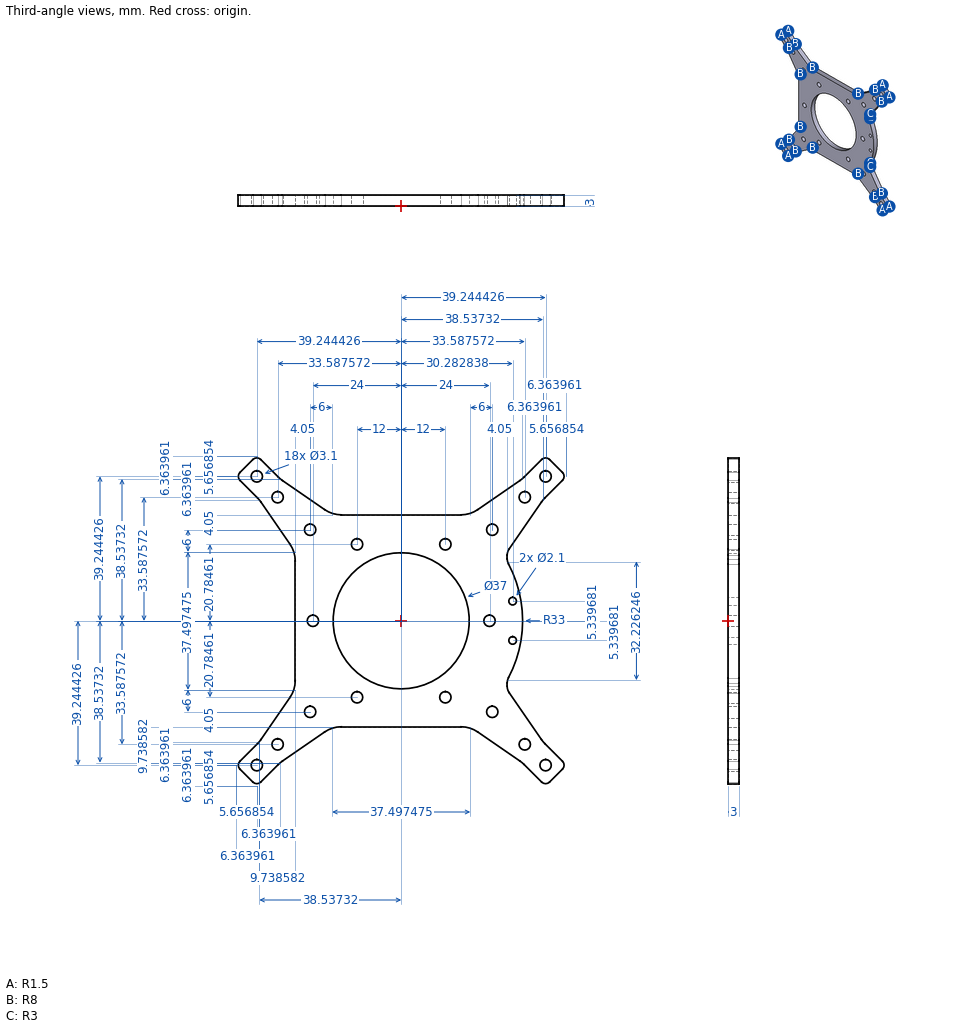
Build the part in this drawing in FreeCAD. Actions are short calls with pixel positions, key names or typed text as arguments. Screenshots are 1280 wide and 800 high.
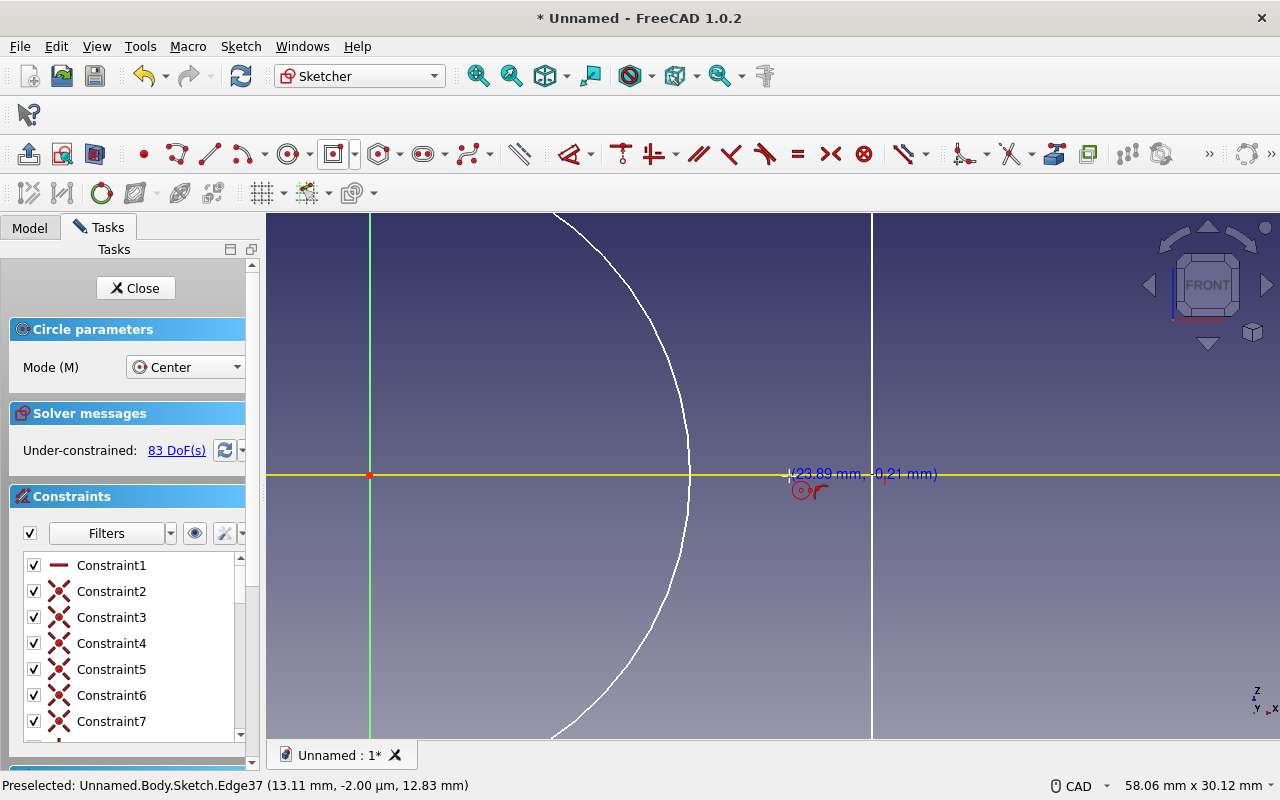
scroll(789, 476, down, 8)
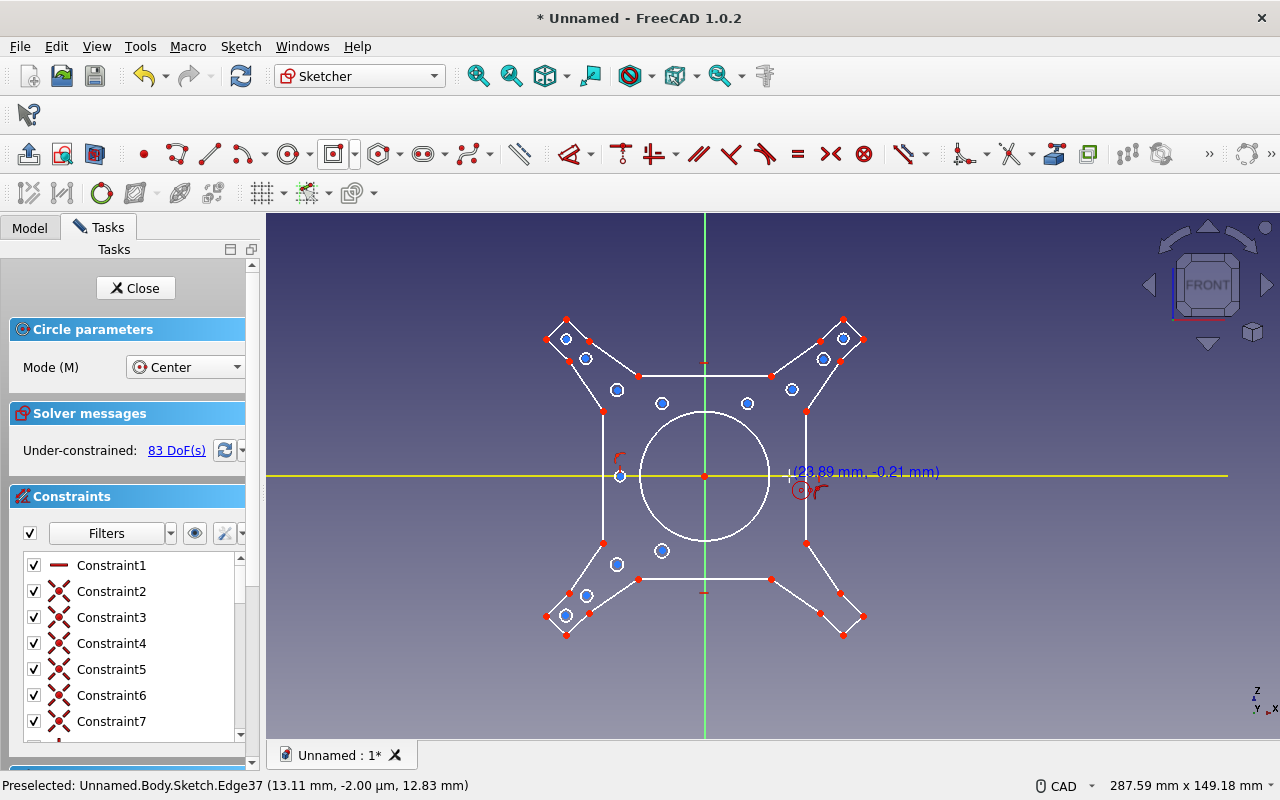
click(789, 476)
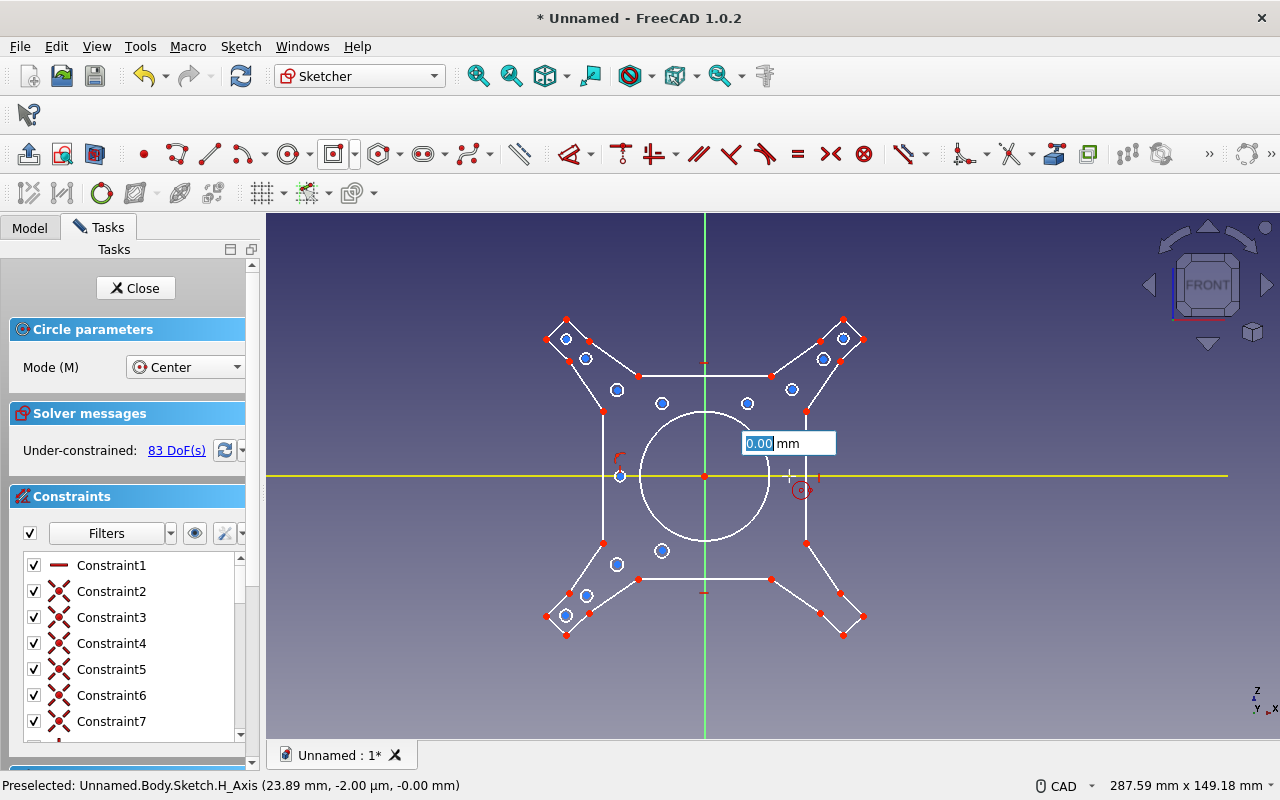
scroll(791, 471, up, 6)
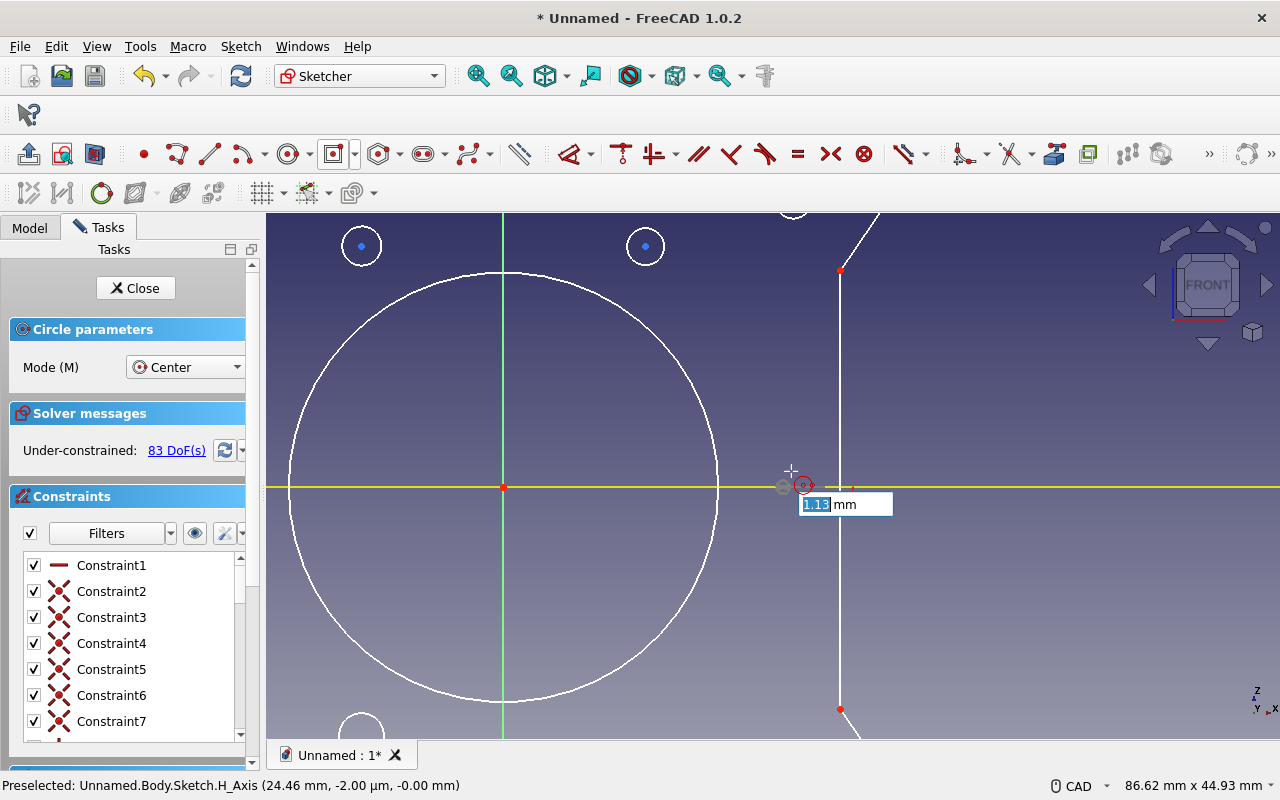
click(791, 470)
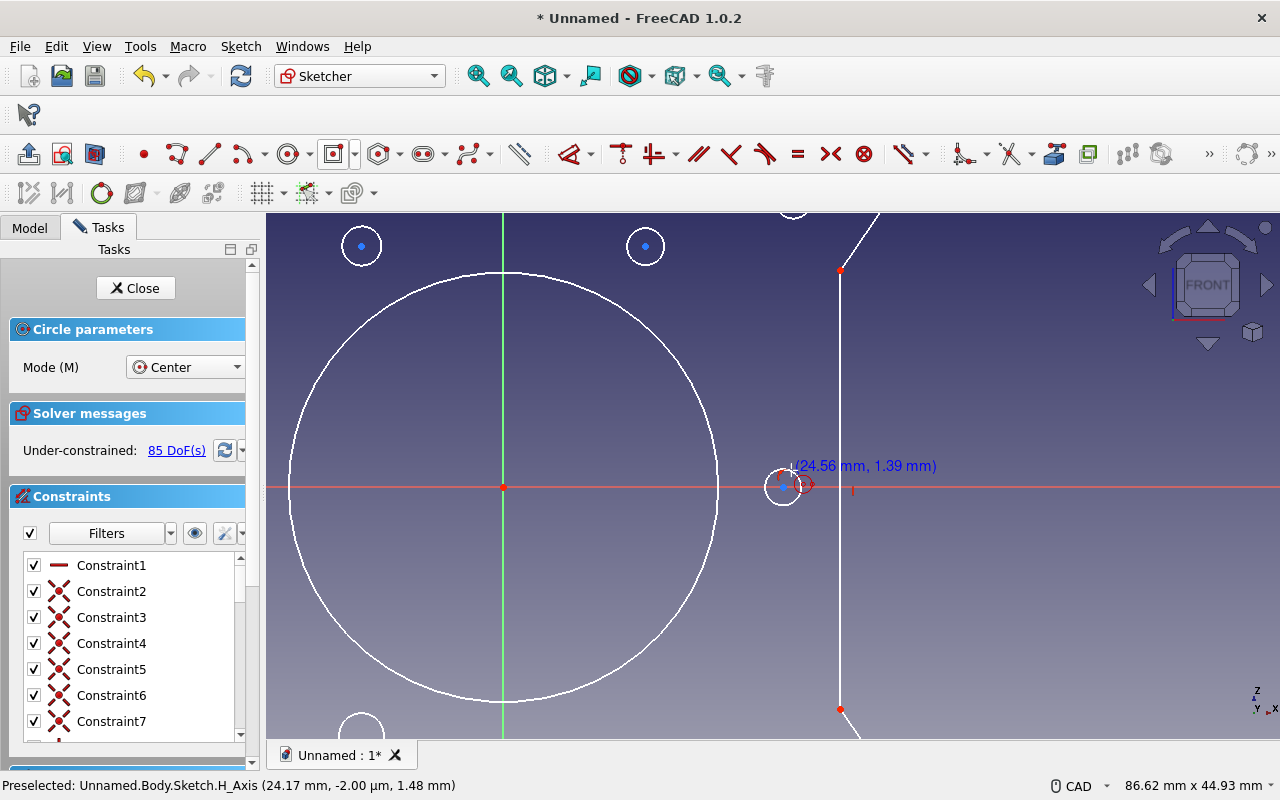
scroll(791, 471, down, 6)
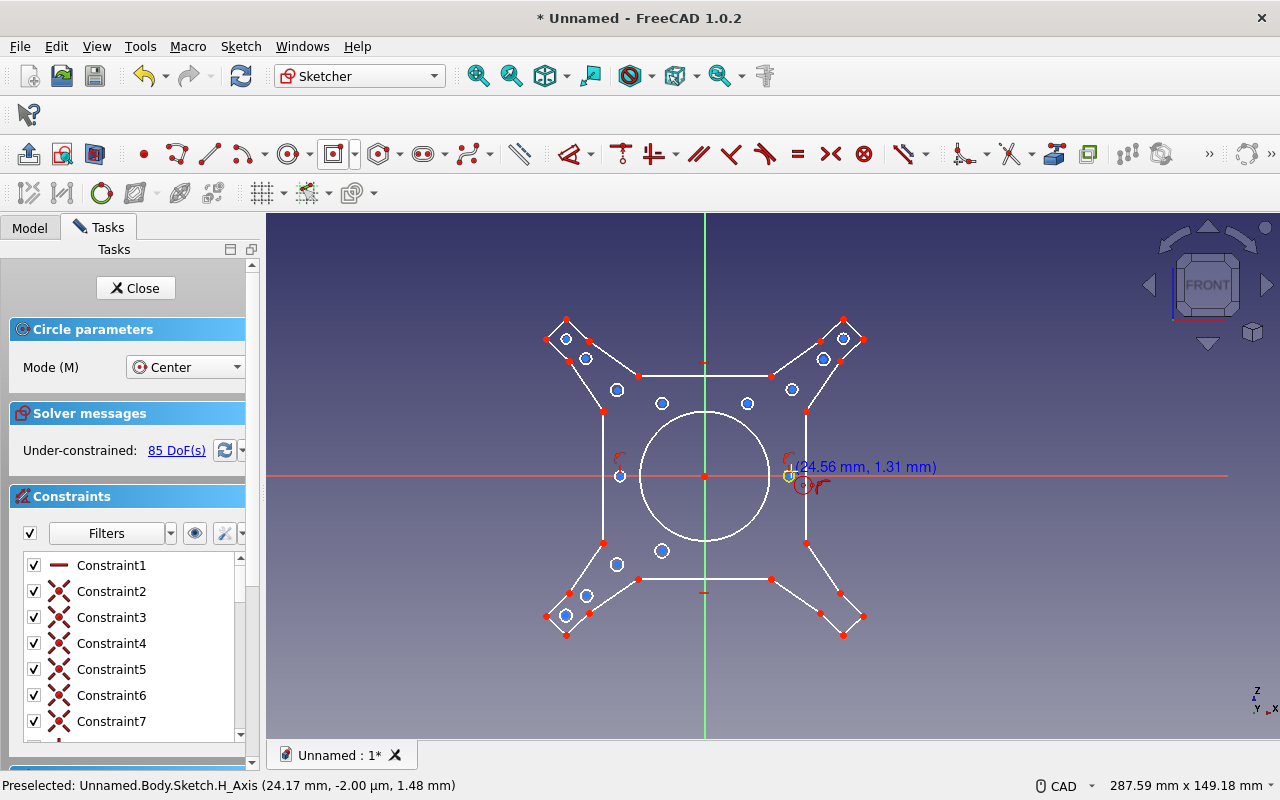
scroll(747, 550, up, 8)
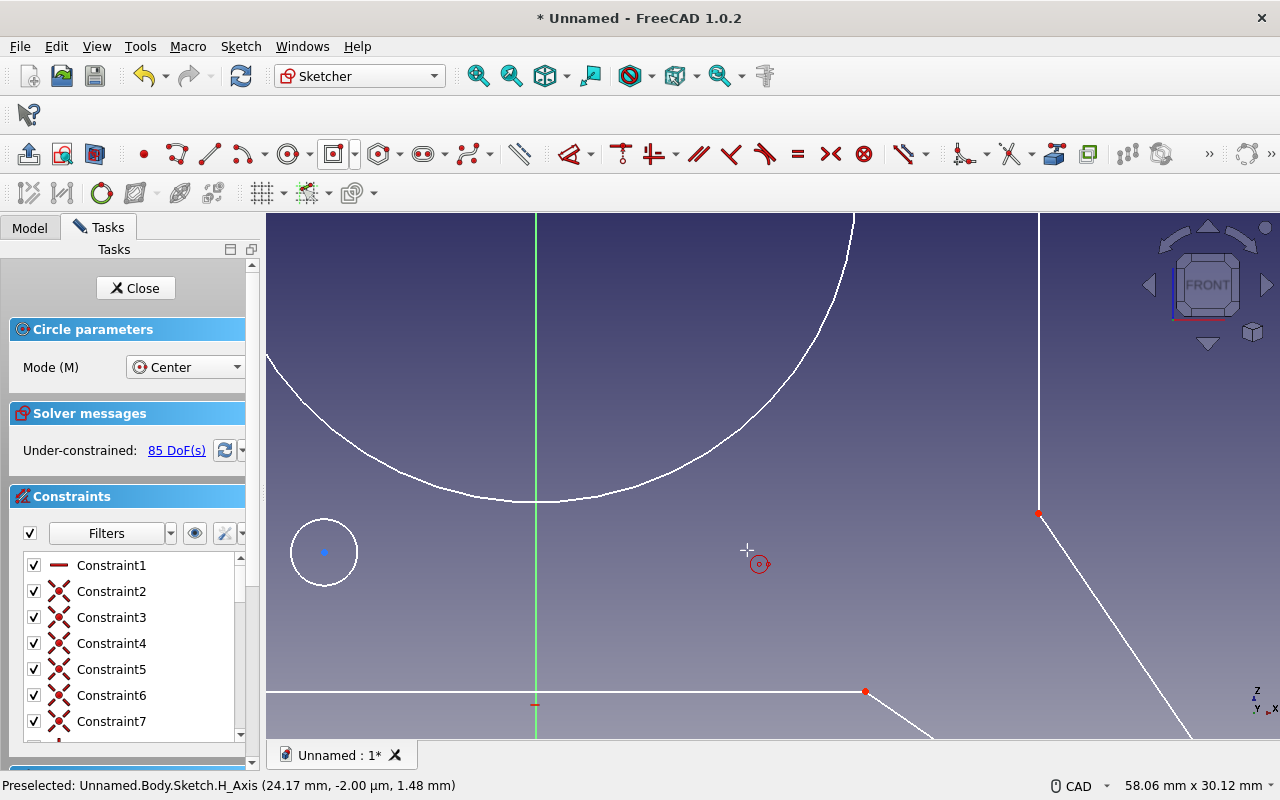
scroll(747, 550, down, 8)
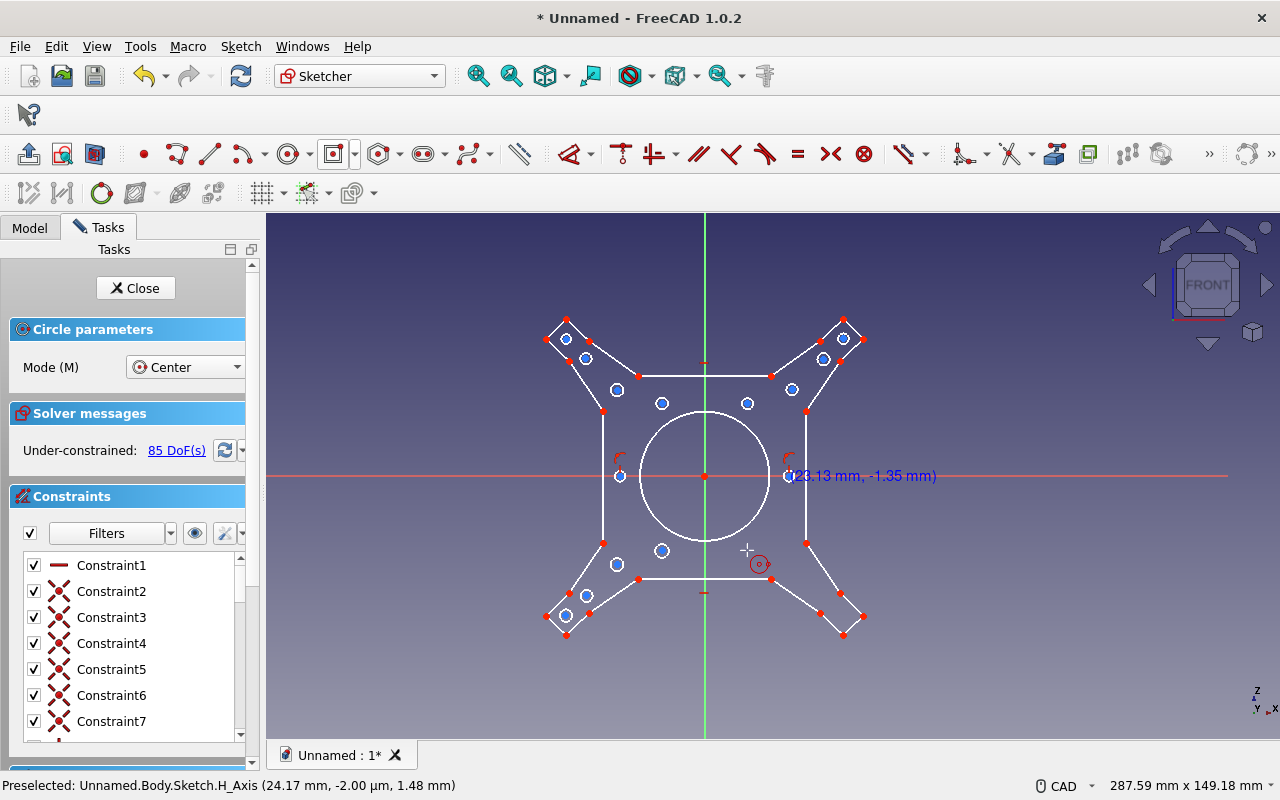
click(747, 550)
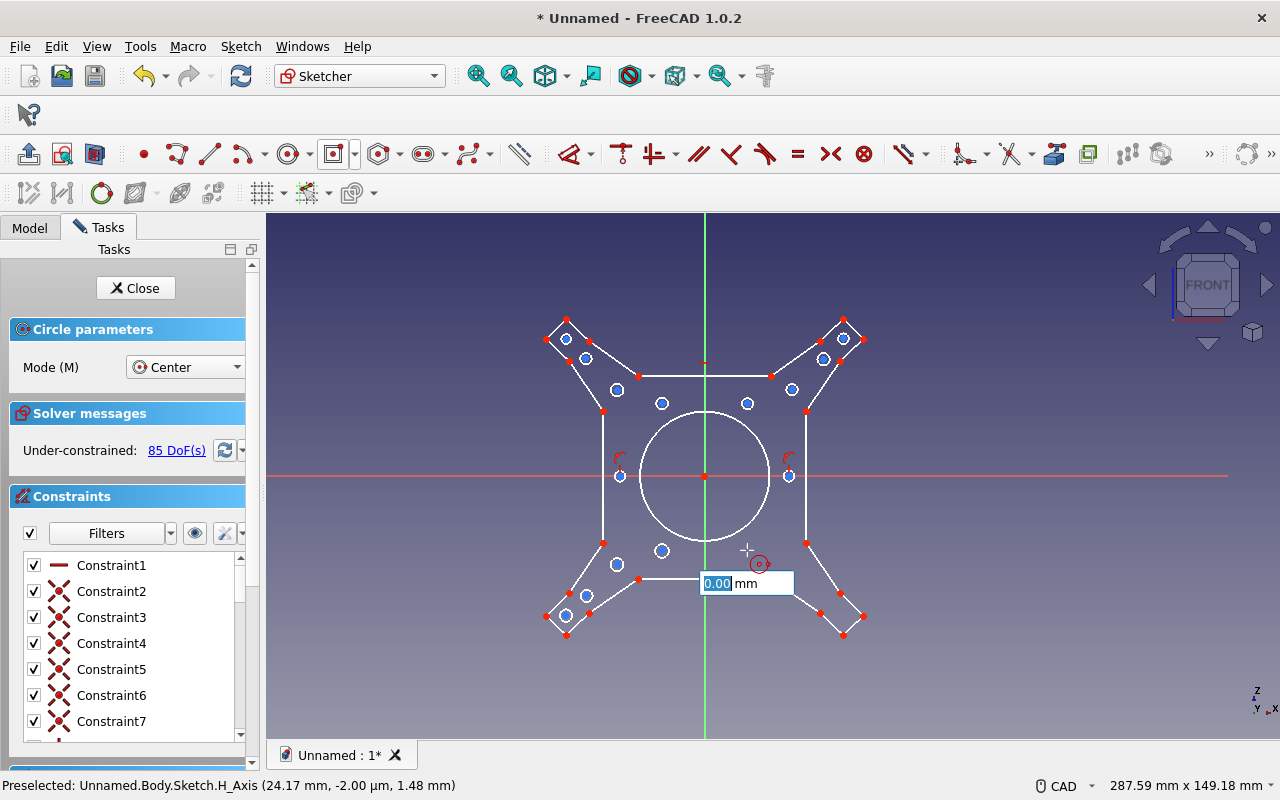
scroll(751, 546, up, 6)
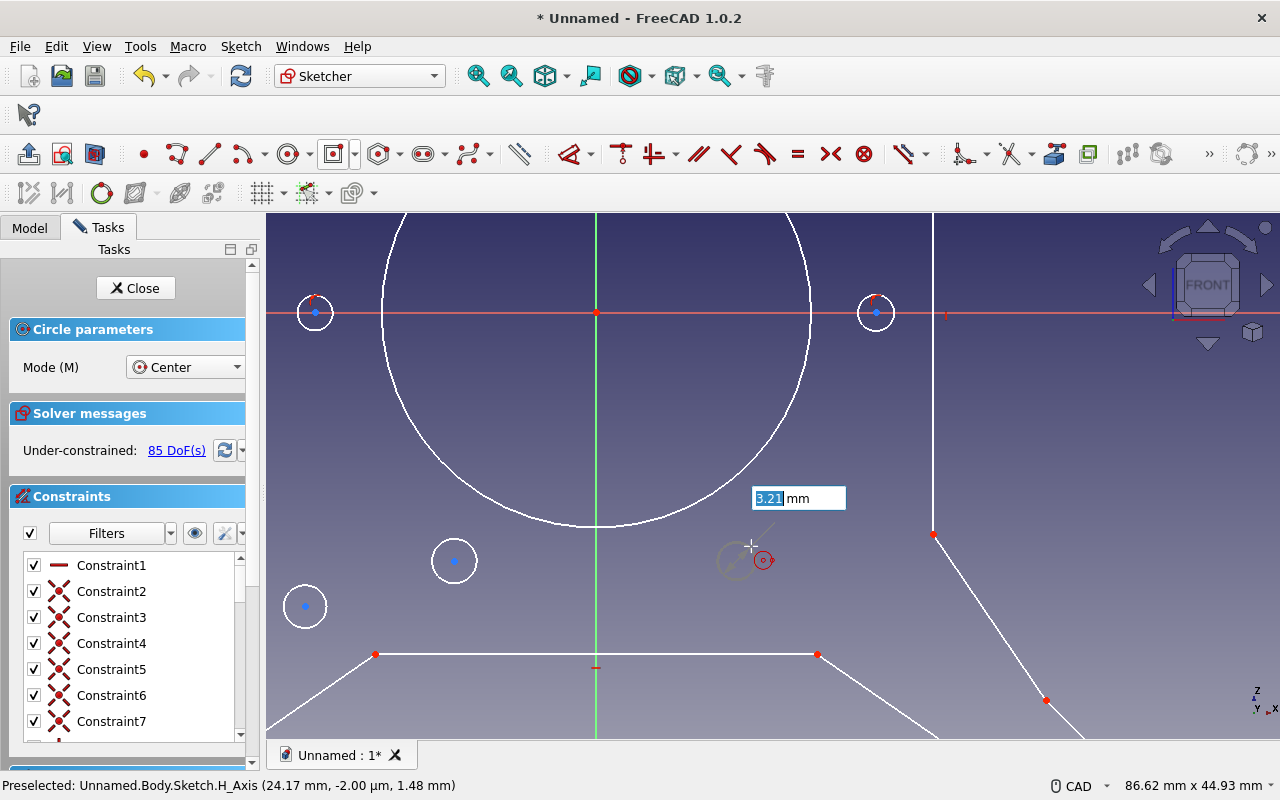
click(750, 543)